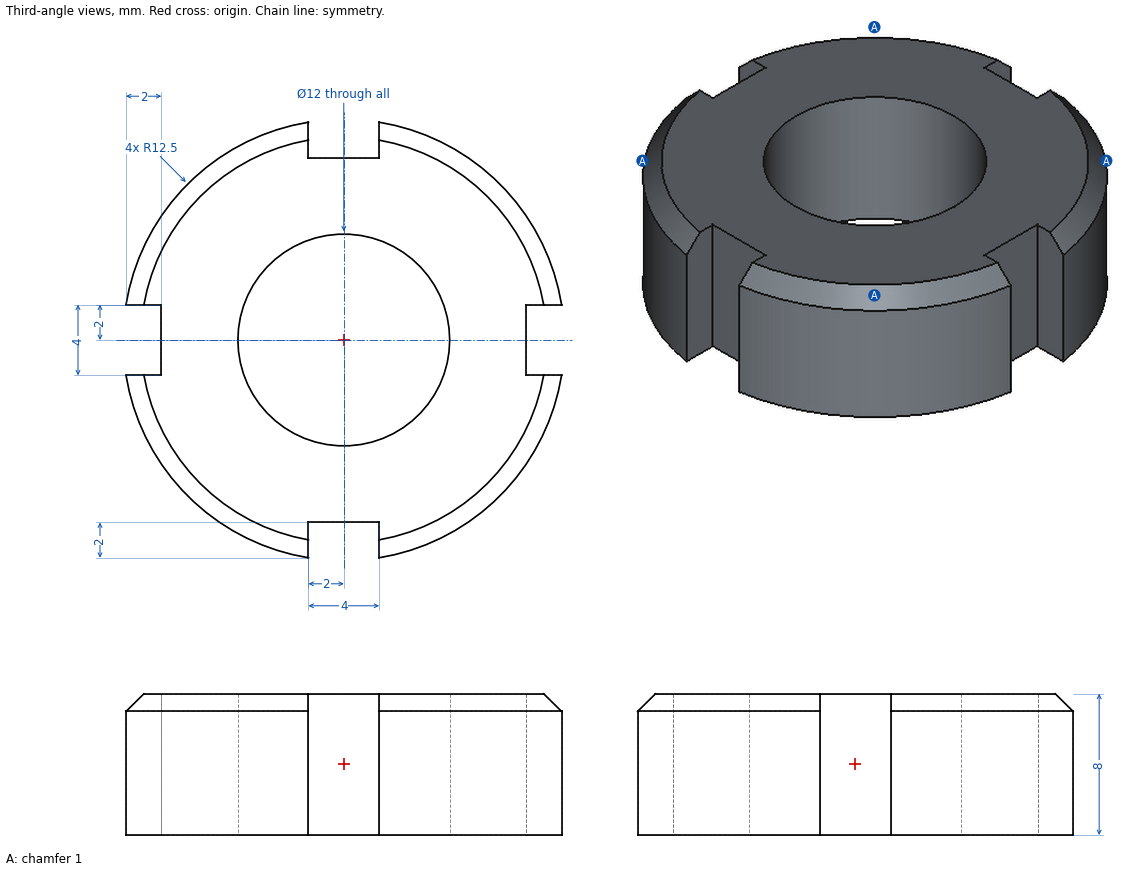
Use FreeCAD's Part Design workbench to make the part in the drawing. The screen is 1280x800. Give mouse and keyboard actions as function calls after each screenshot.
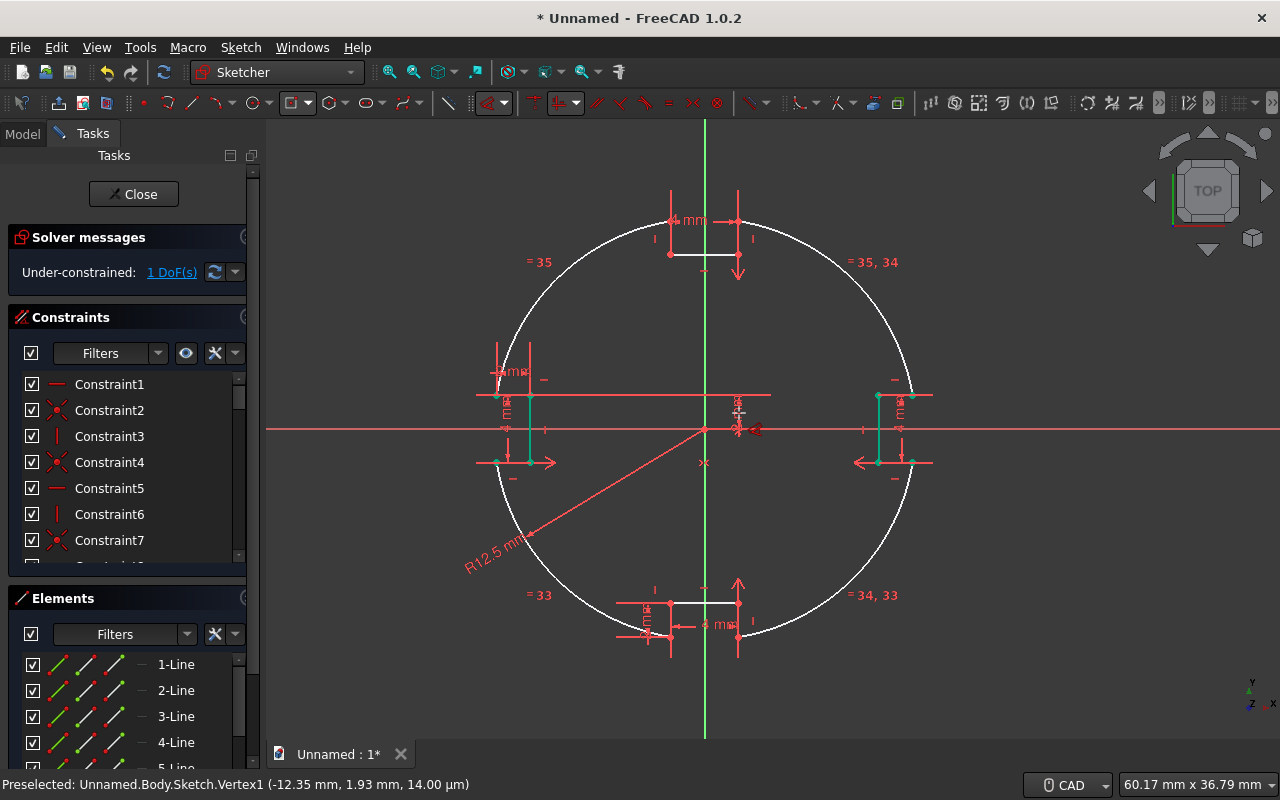
click(671, 637)
click(688, 671)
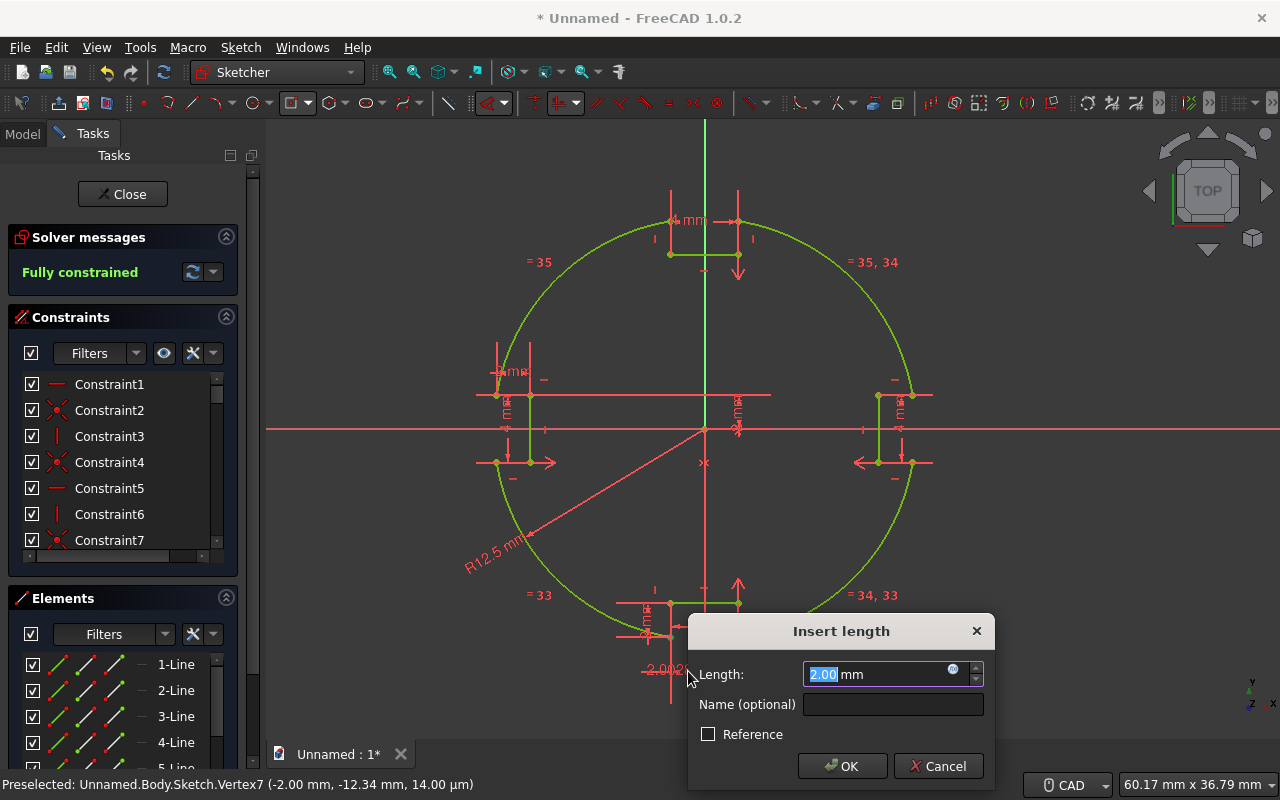
text(2)
key(Return)
key(Escape)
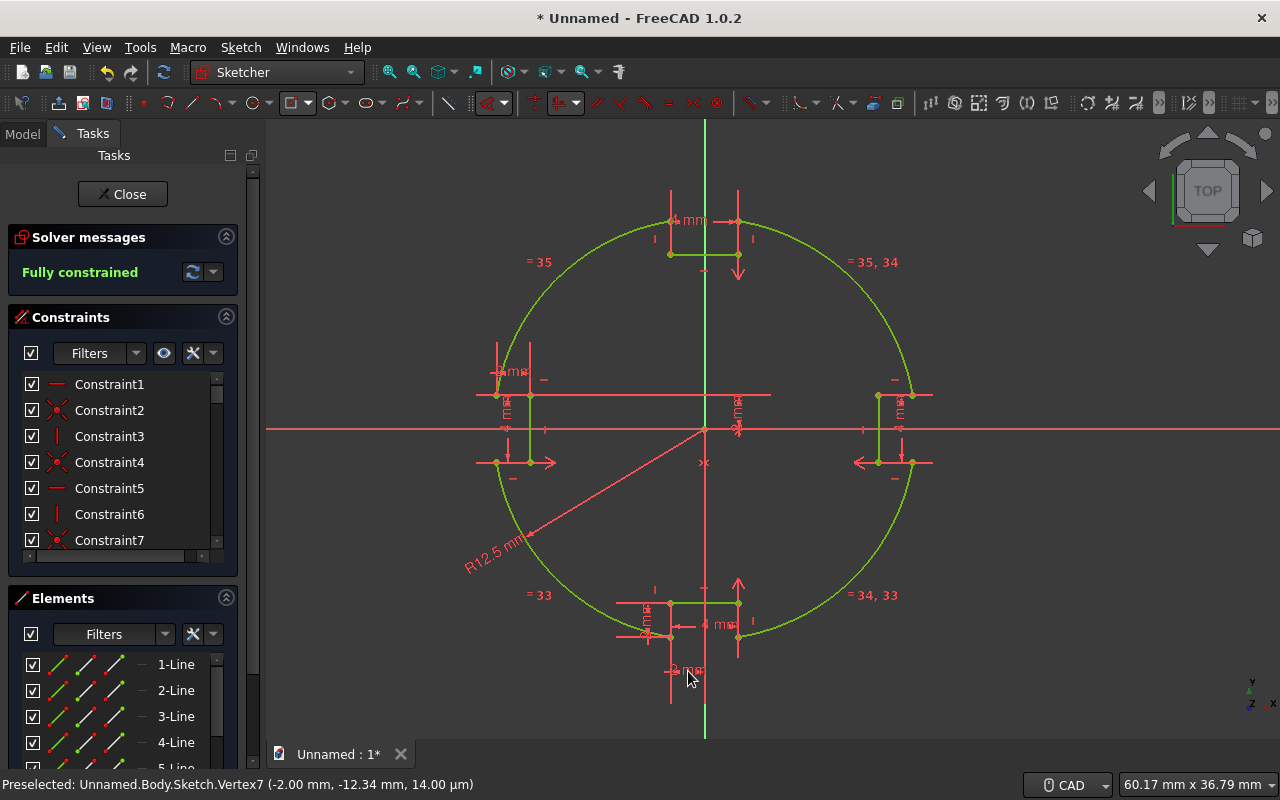
click(123, 194)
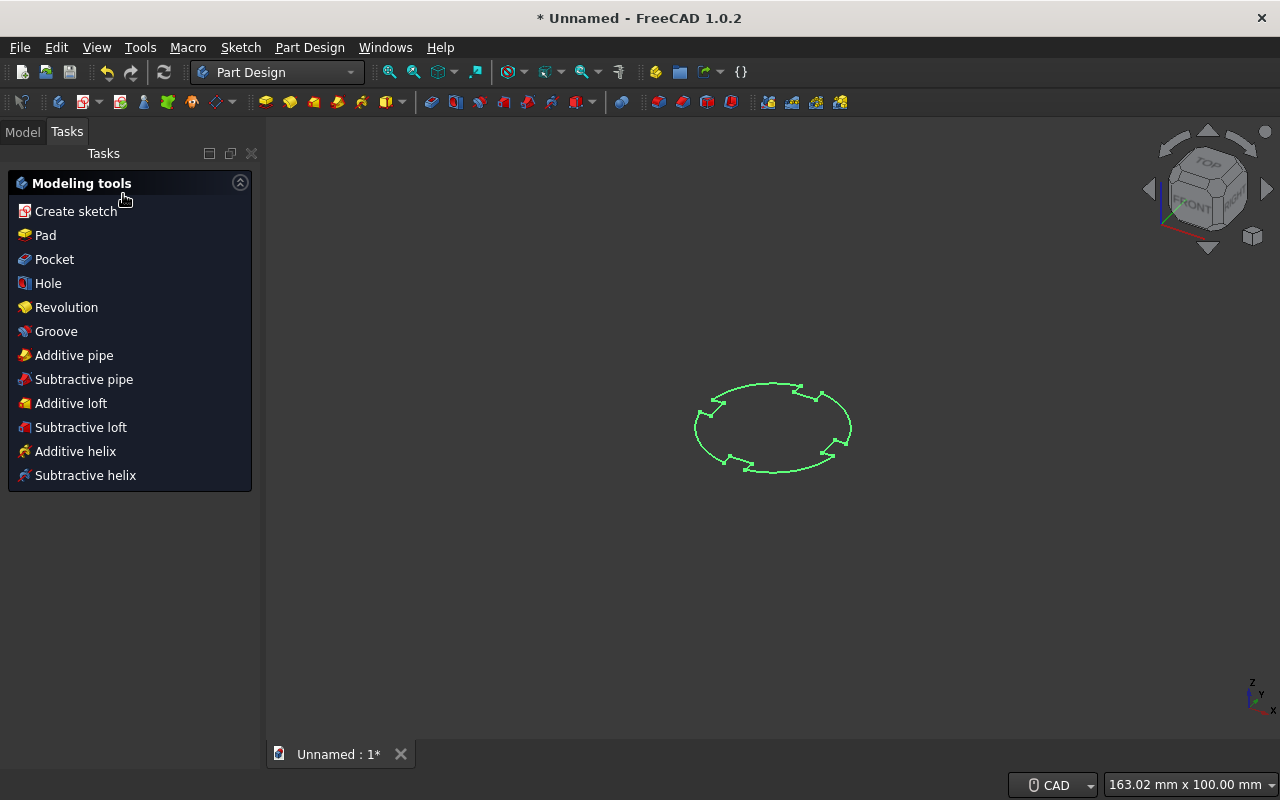
click(266, 102)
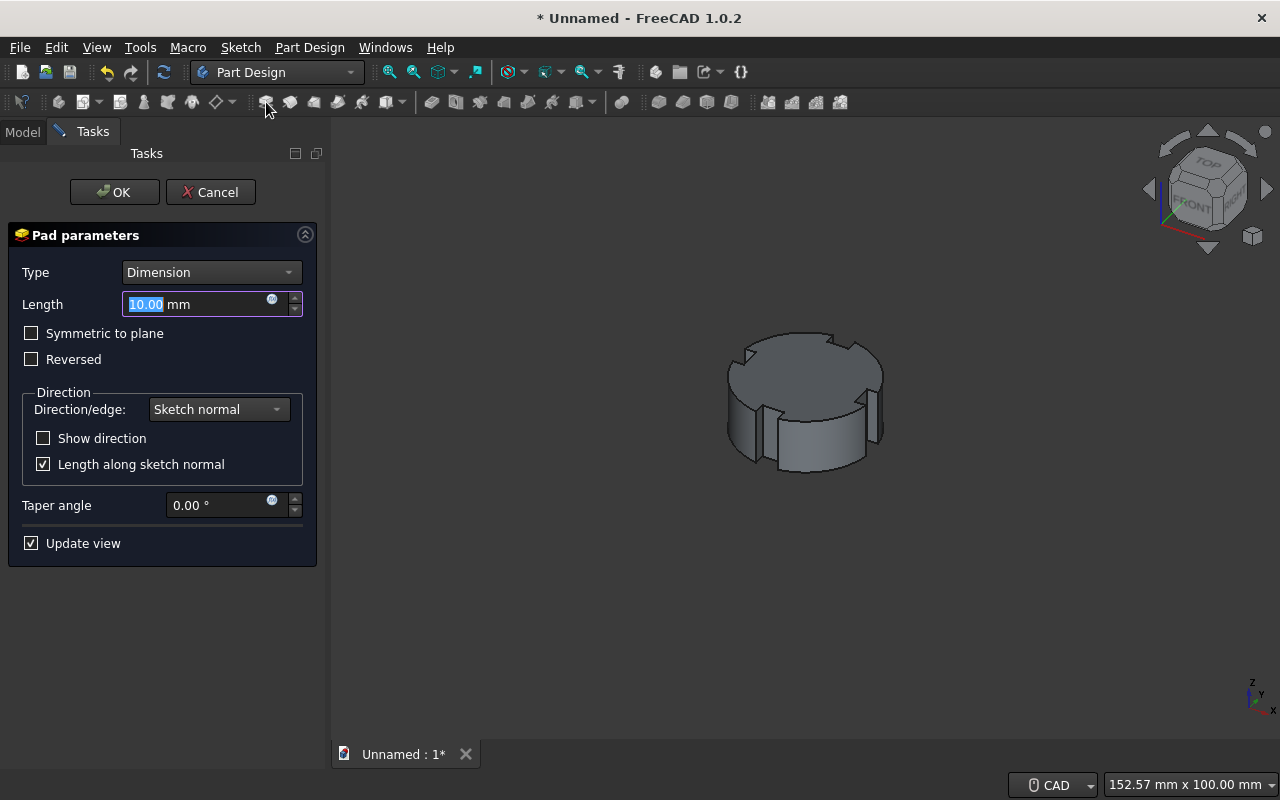
text(8)
key(Tab)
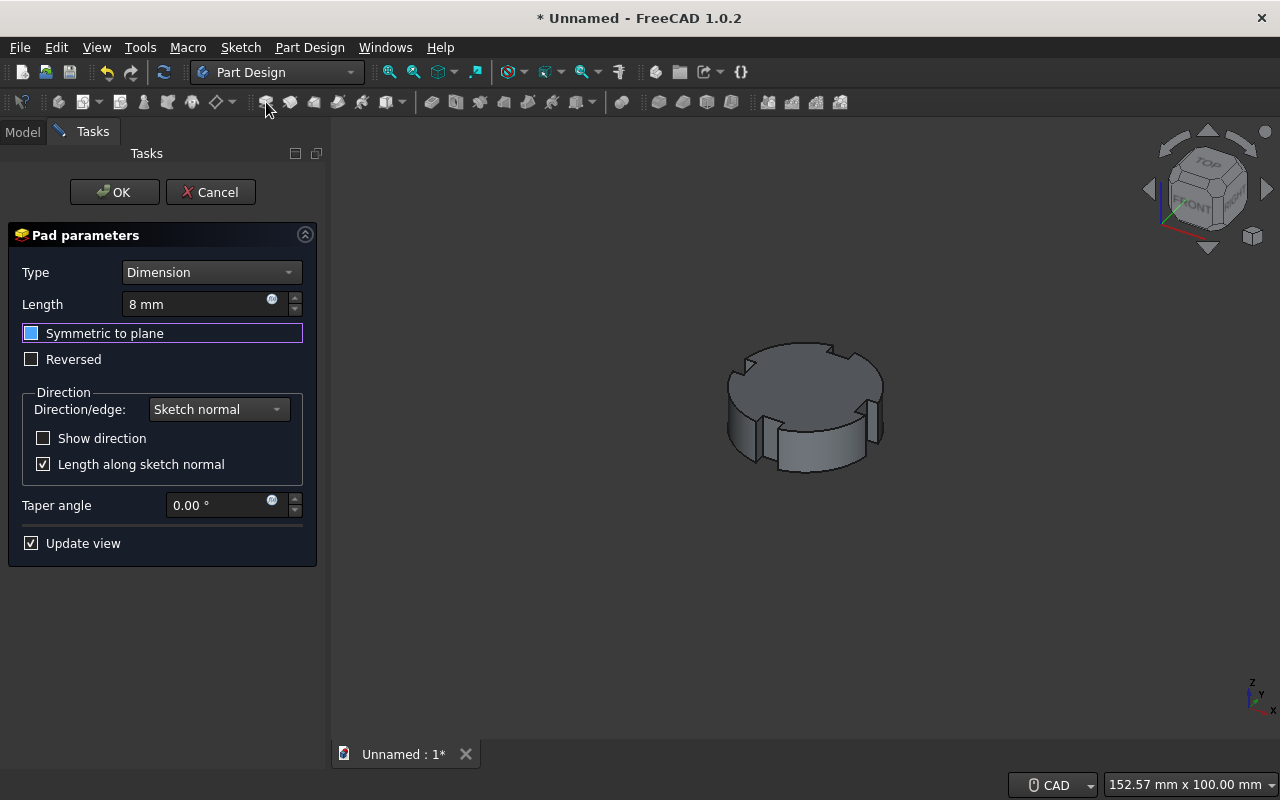
click(30, 333)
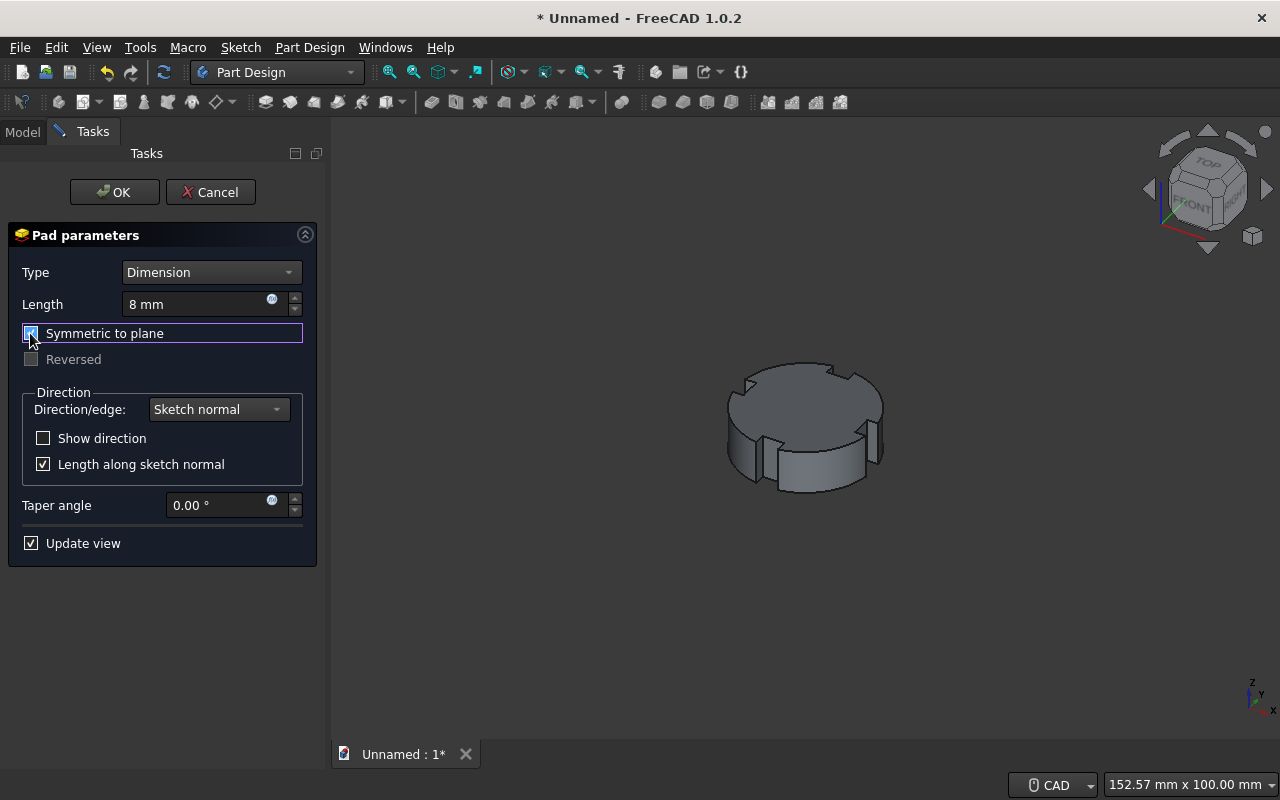
click(115, 192)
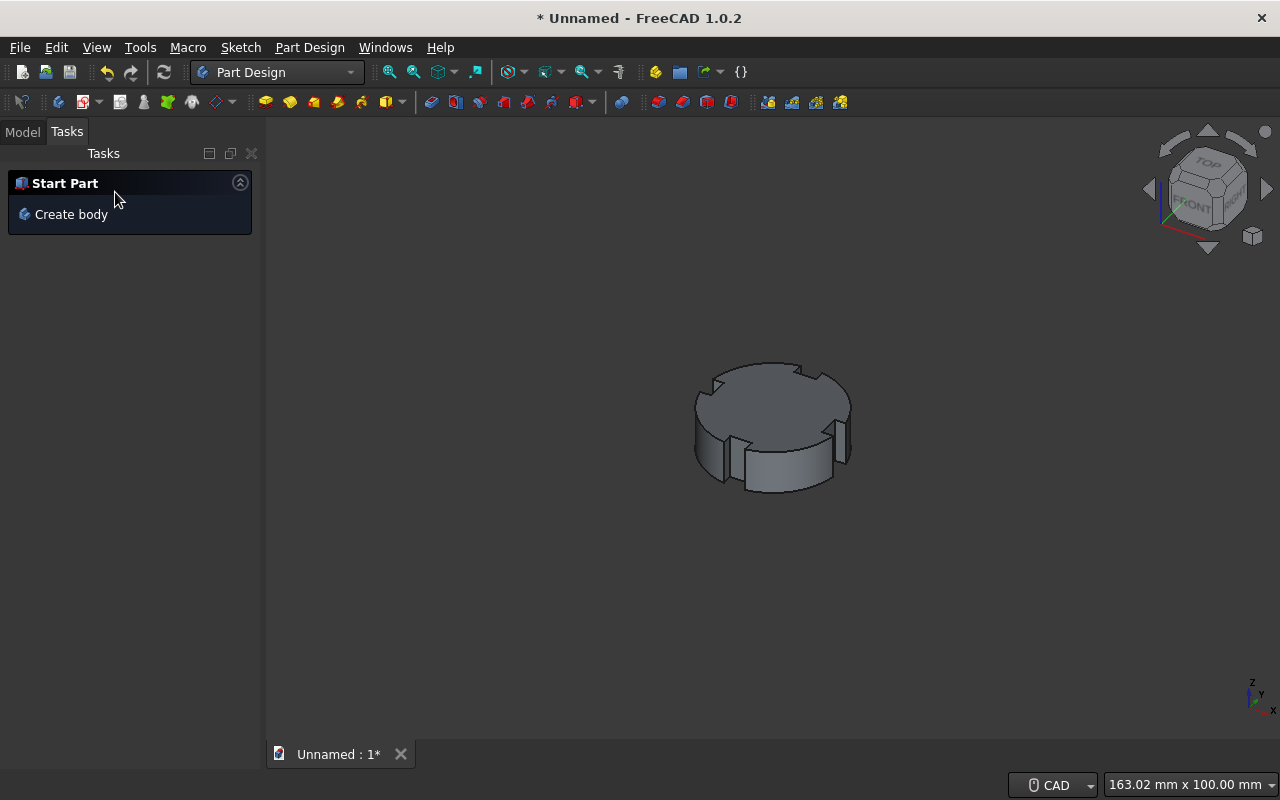
key(v)
key(f)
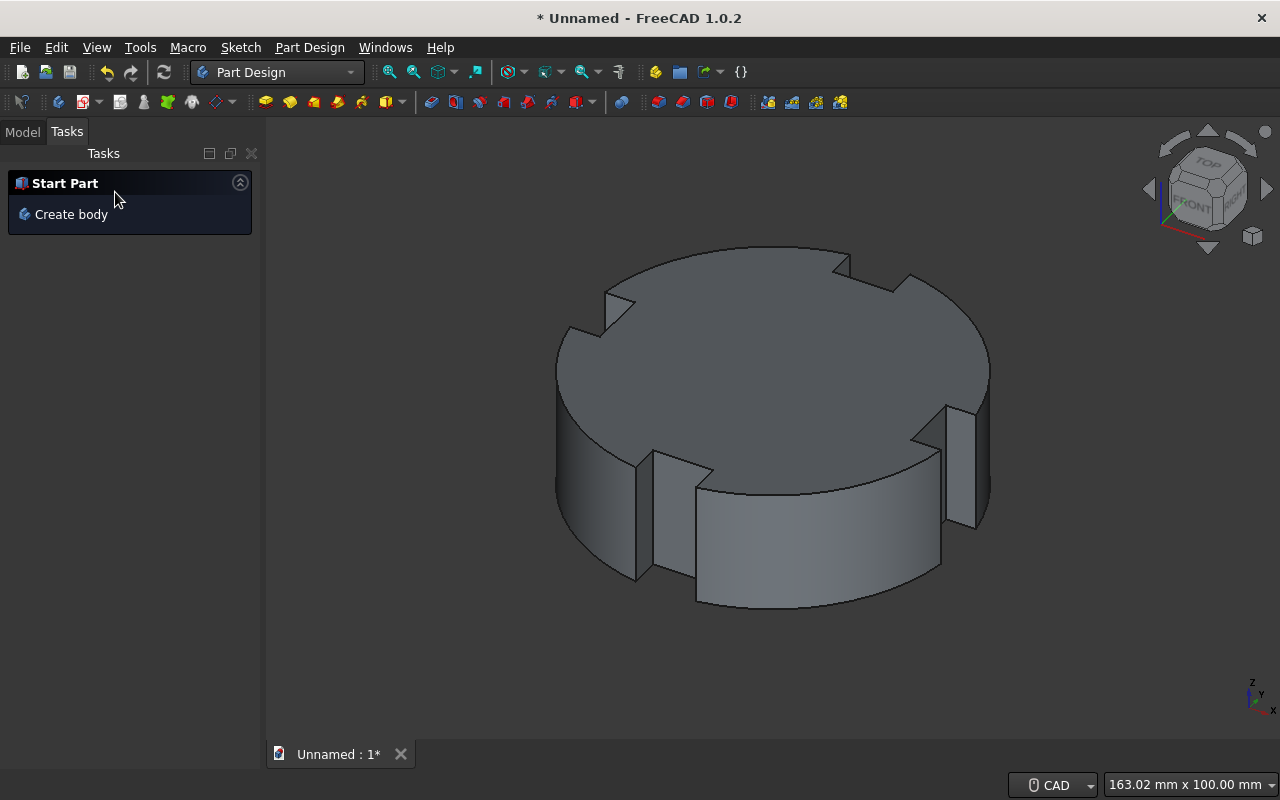
click(773, 370)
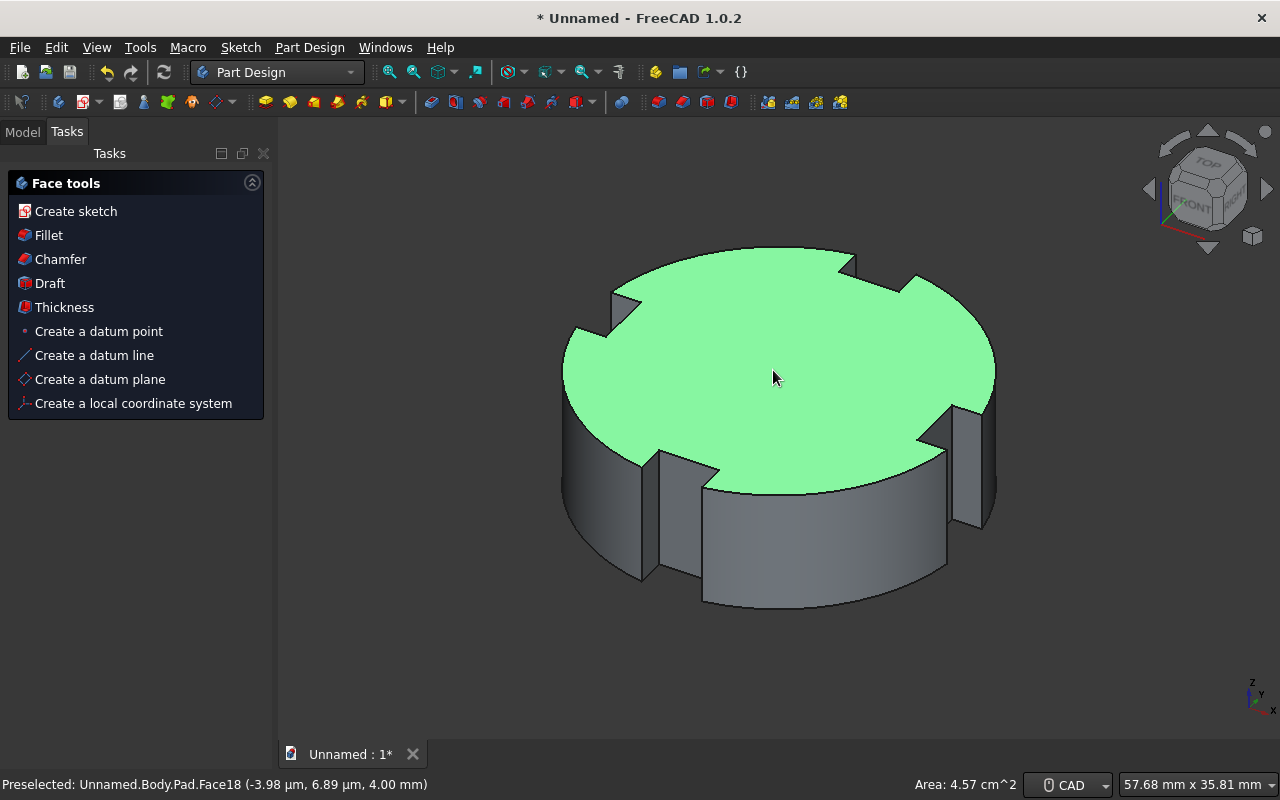
click(84, 102)